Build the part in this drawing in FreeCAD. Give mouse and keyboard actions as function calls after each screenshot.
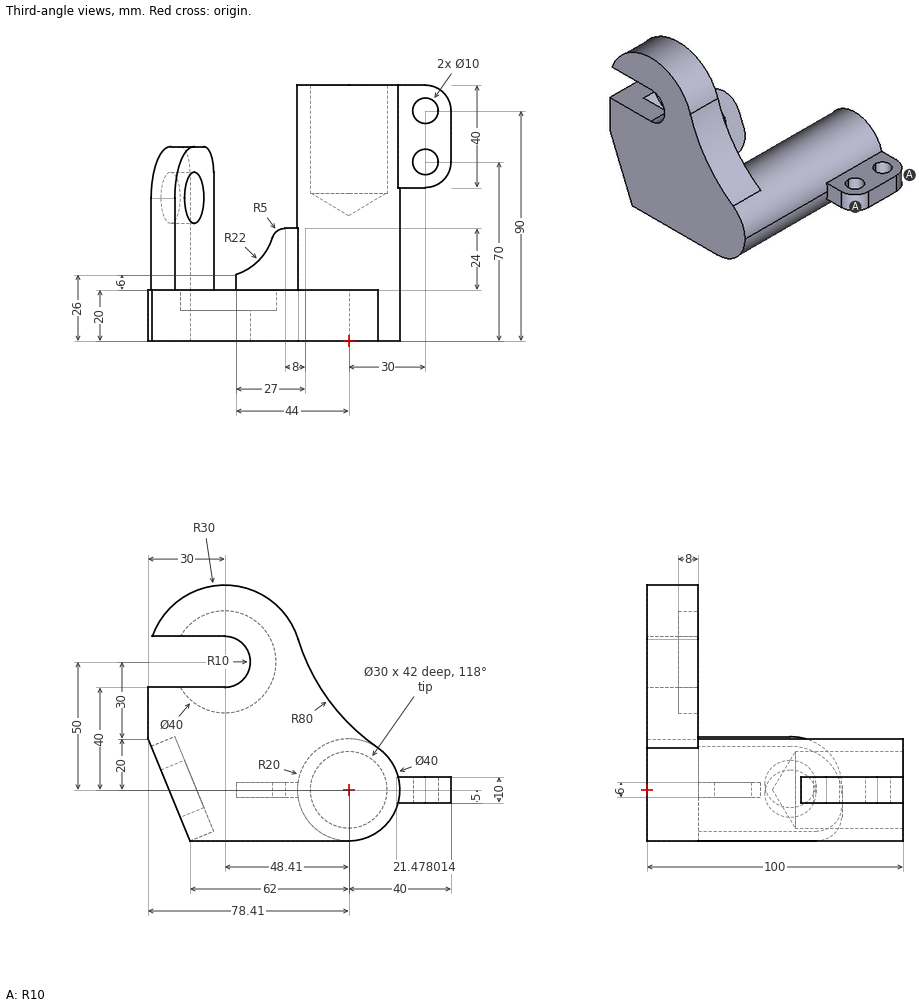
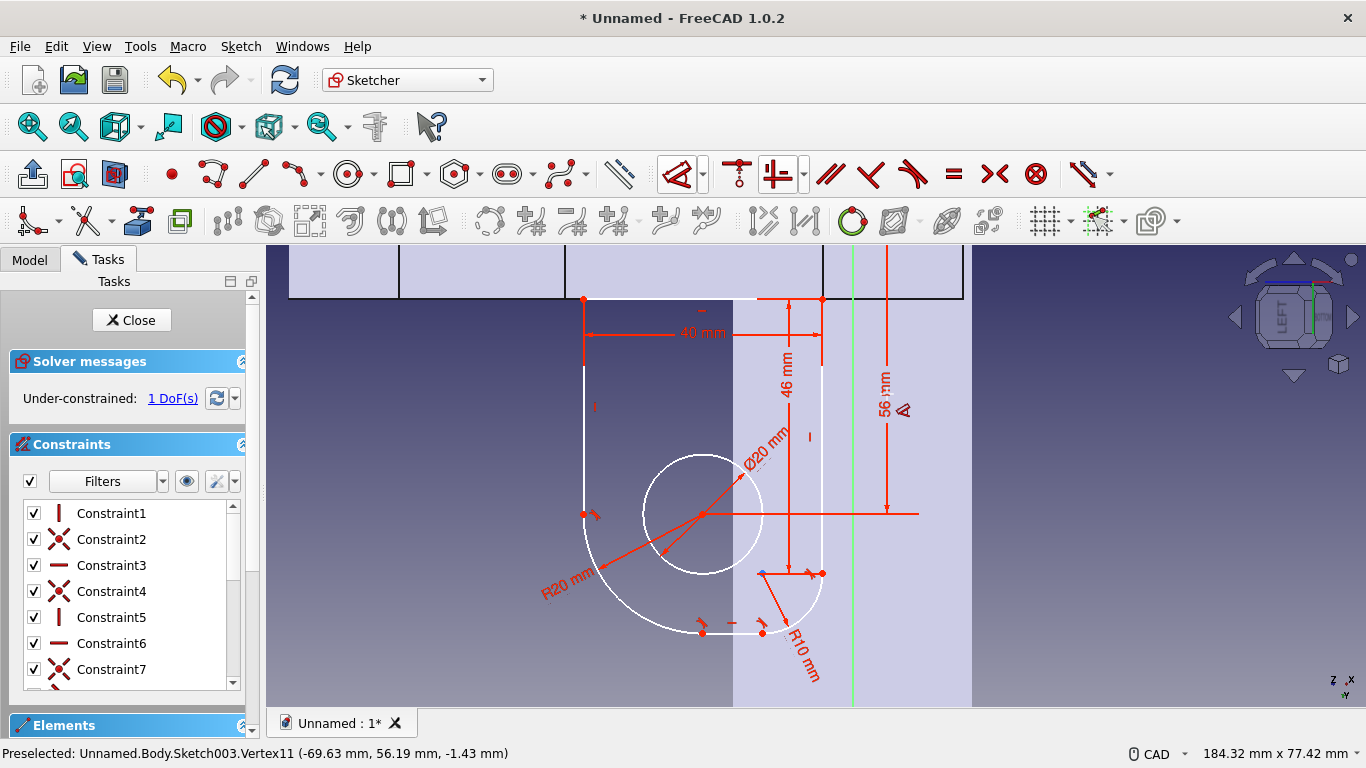
scroll(822, 574, up, 2)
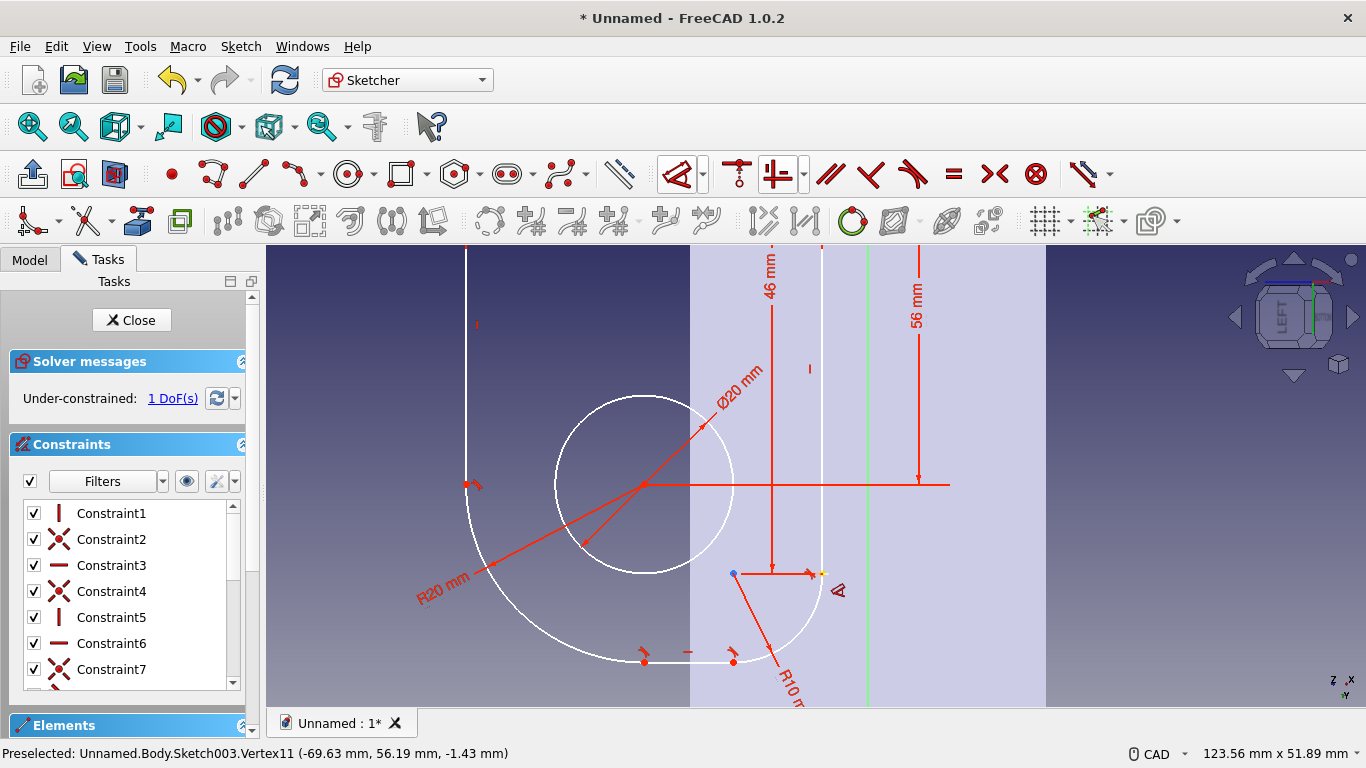
click(822, 574)
click(845, 608)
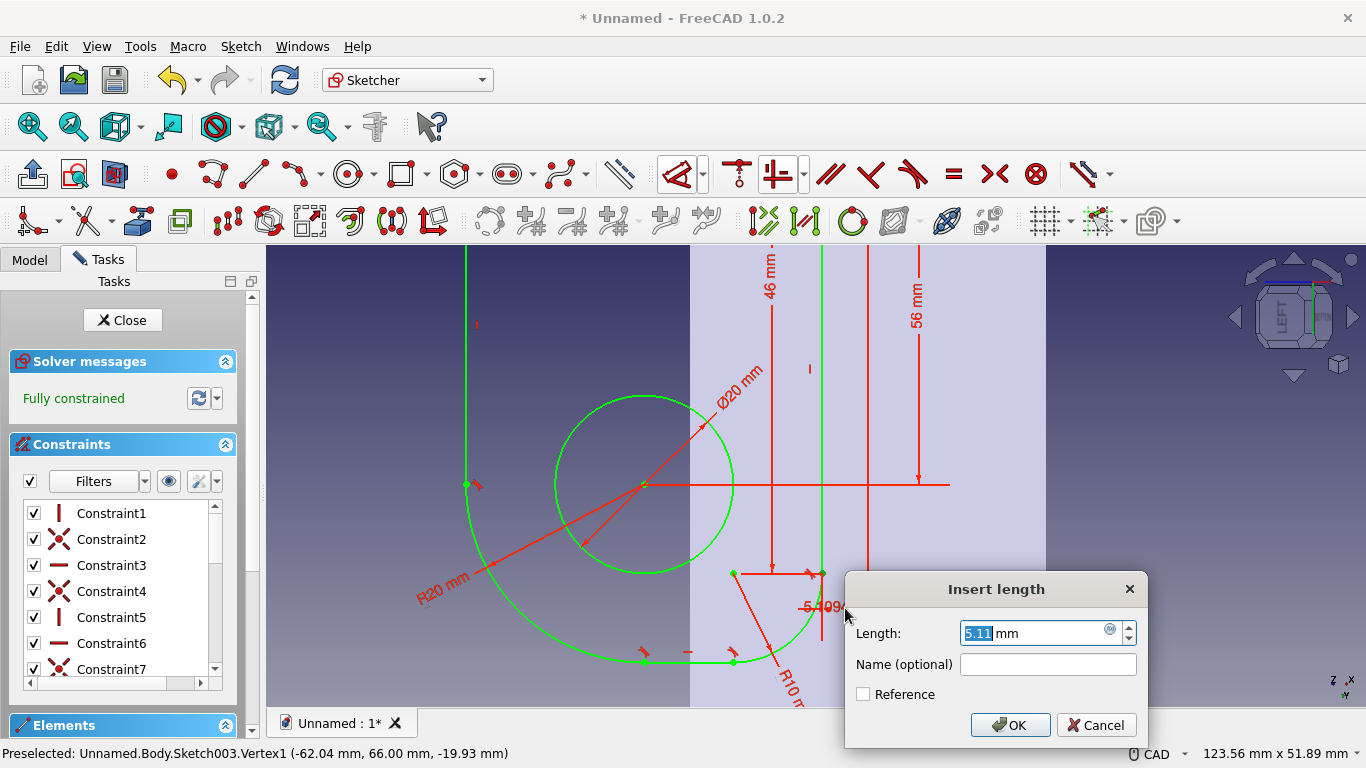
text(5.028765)
key(Return)
key(Escape)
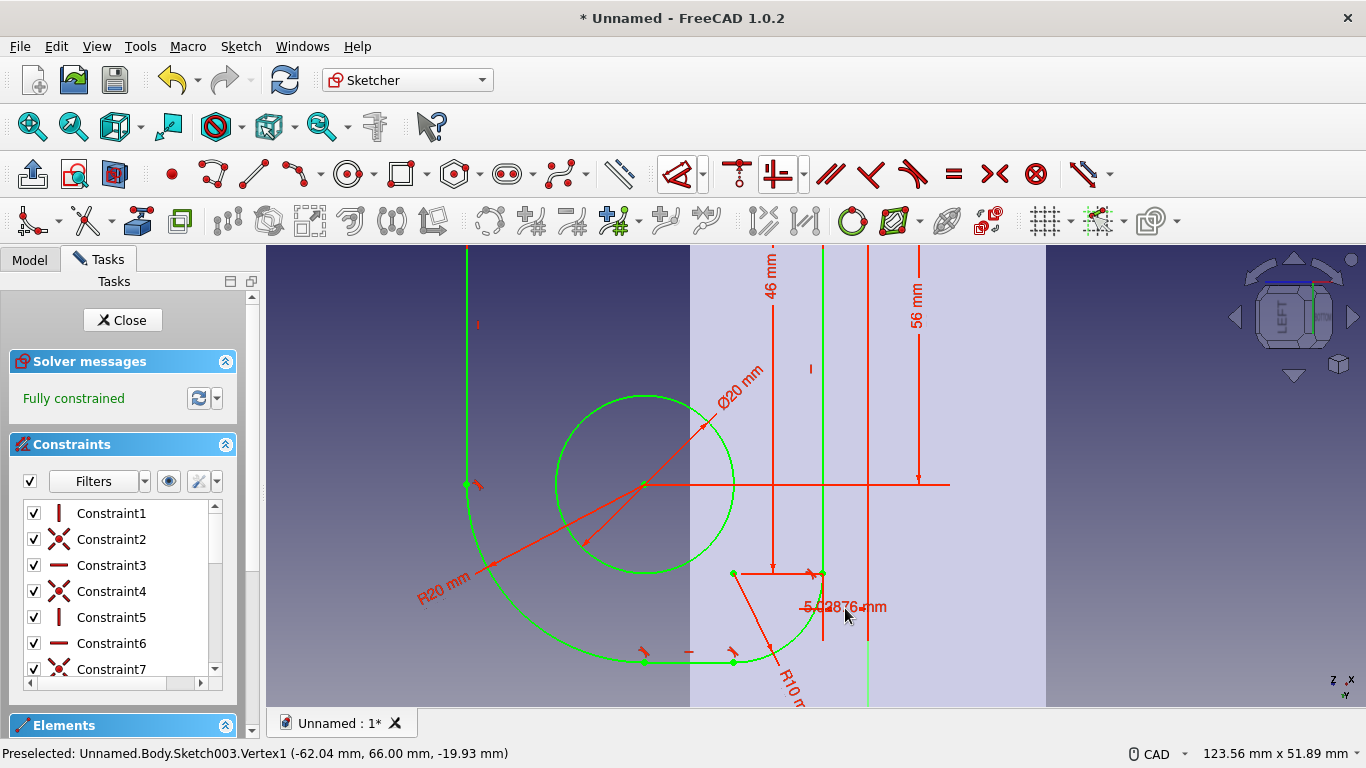
click(123, 320)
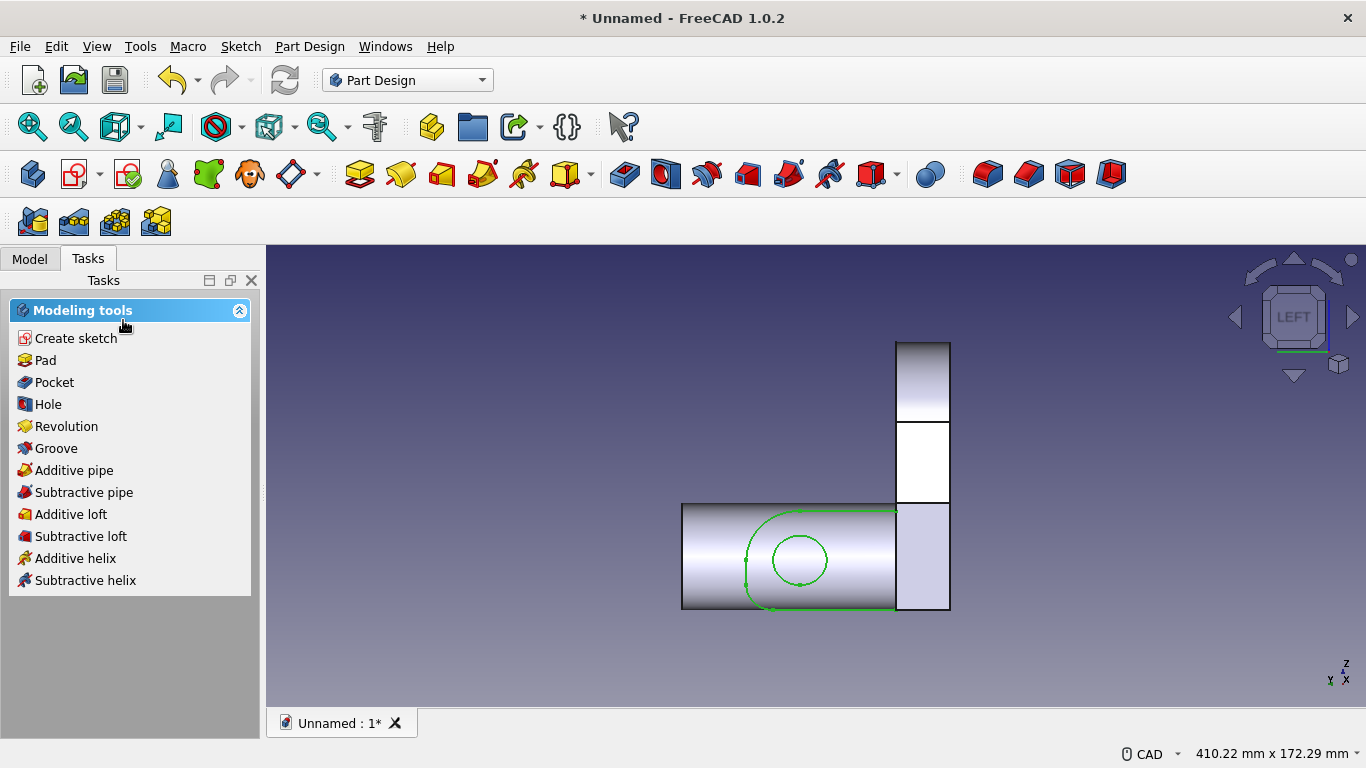
click(360, 174)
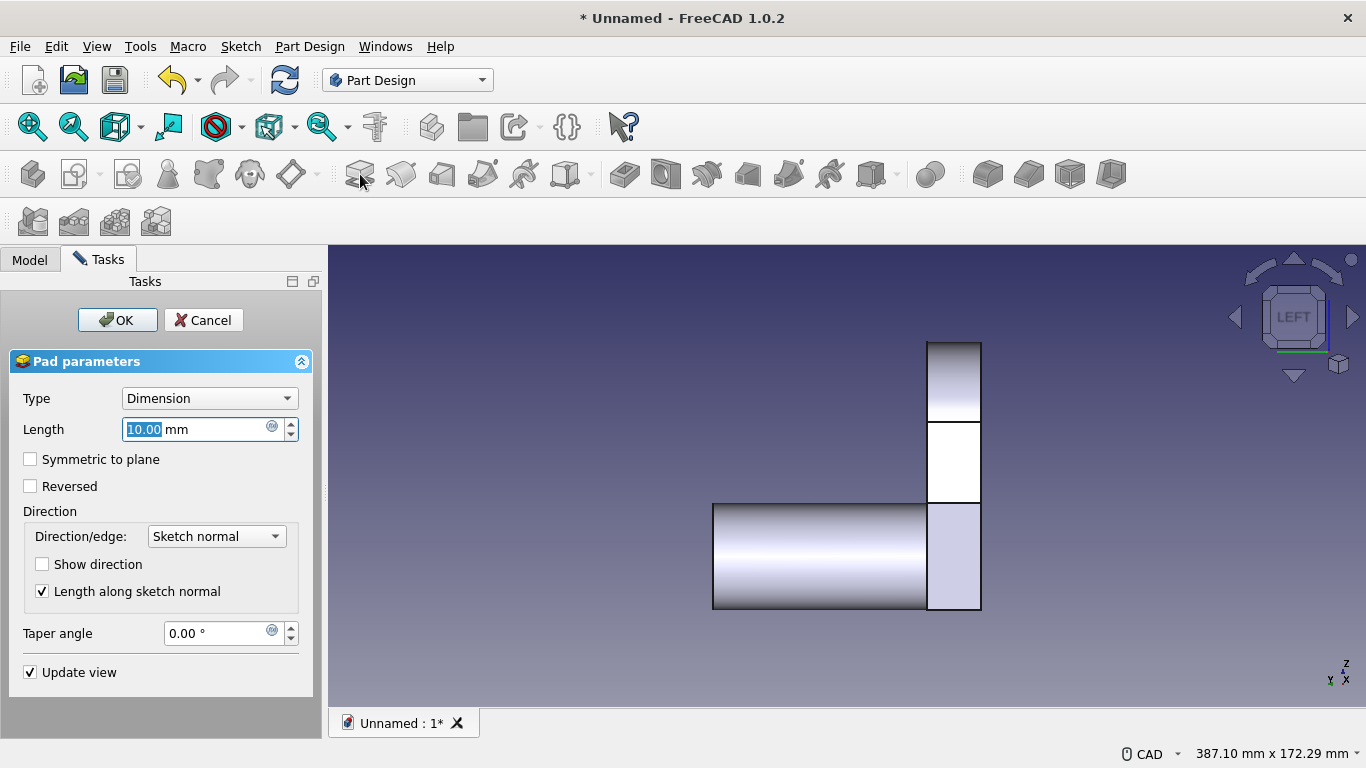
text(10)
key(Tab)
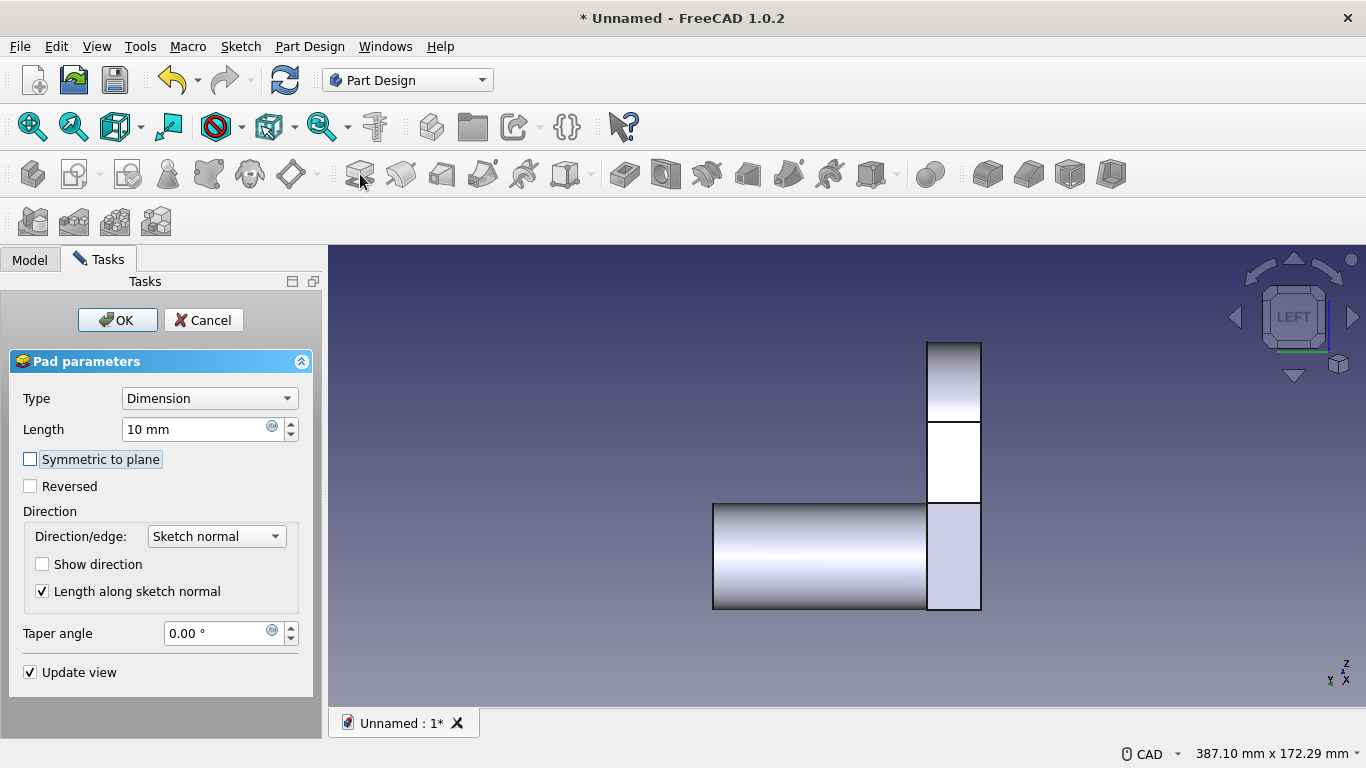
click(31, 486)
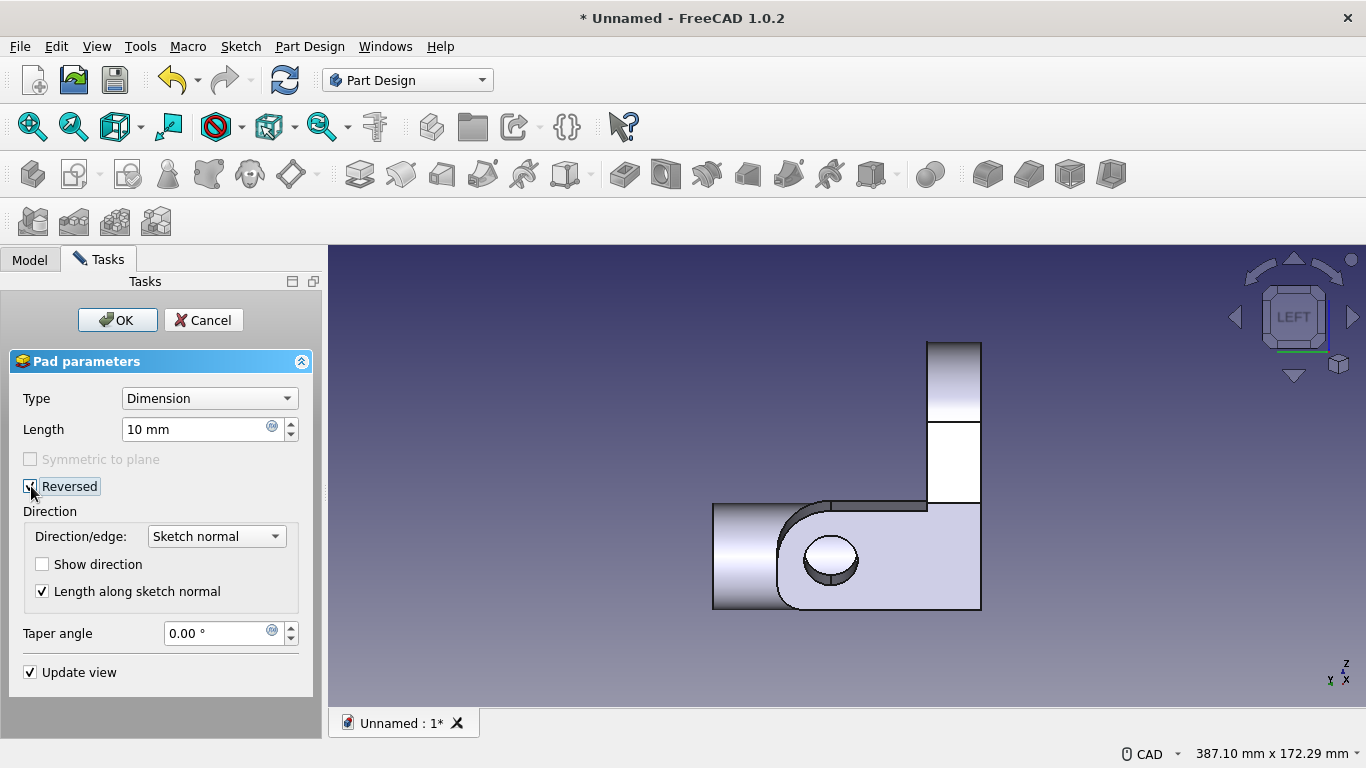
click(118, 320)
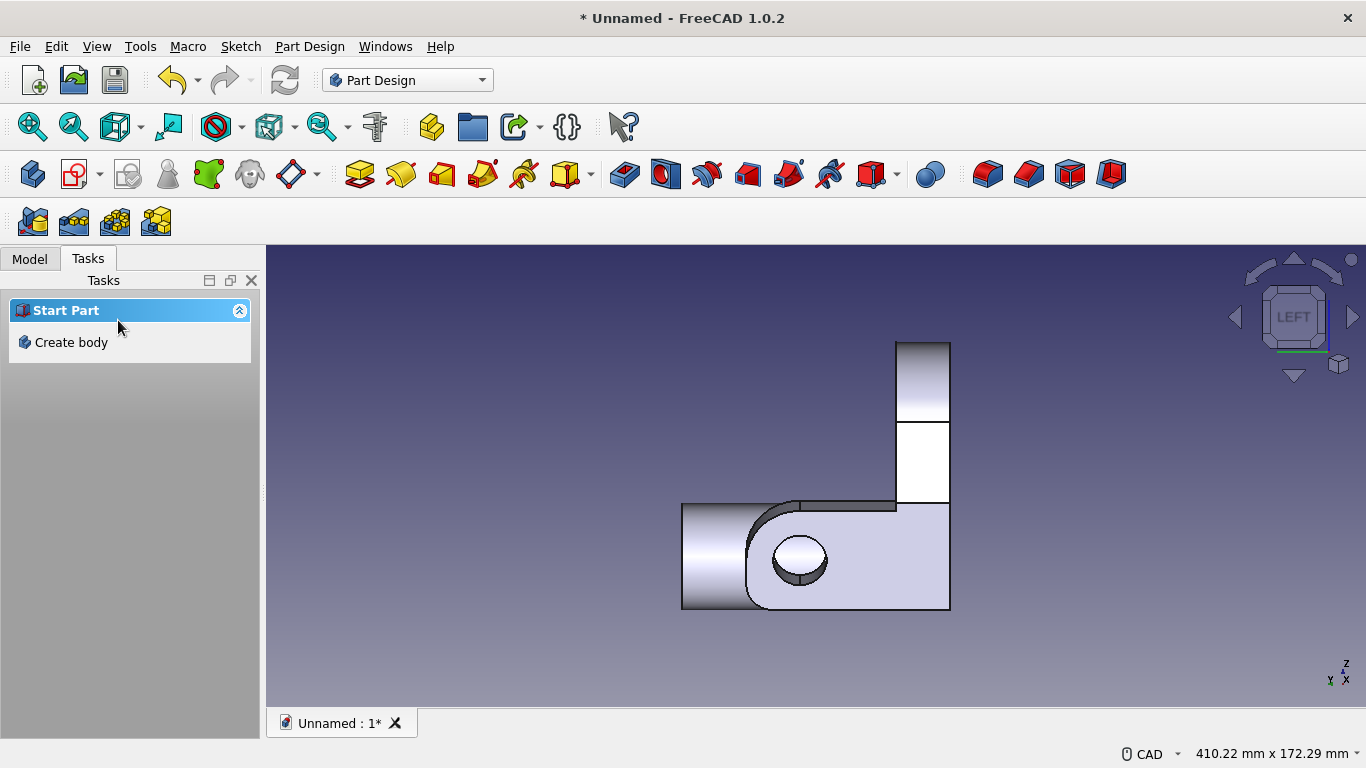
key(4)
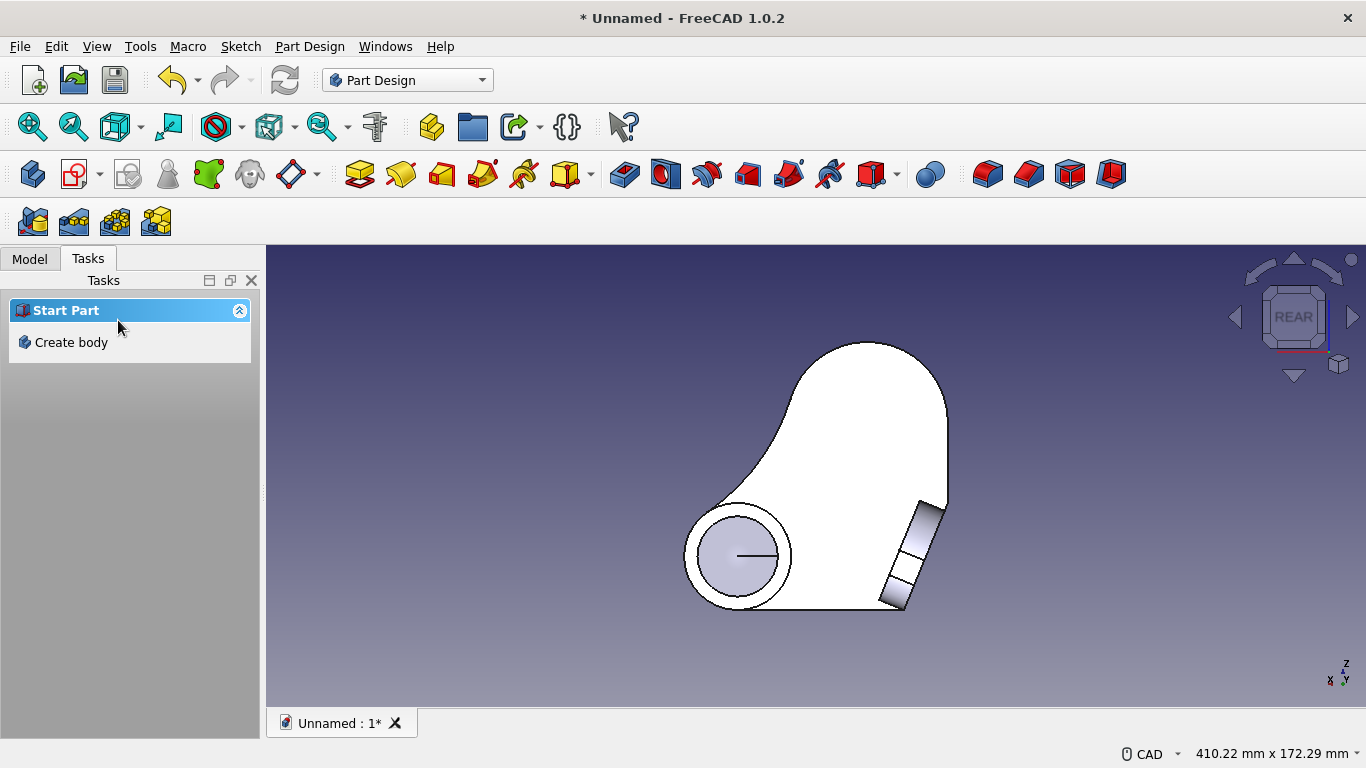
click(862, 437)